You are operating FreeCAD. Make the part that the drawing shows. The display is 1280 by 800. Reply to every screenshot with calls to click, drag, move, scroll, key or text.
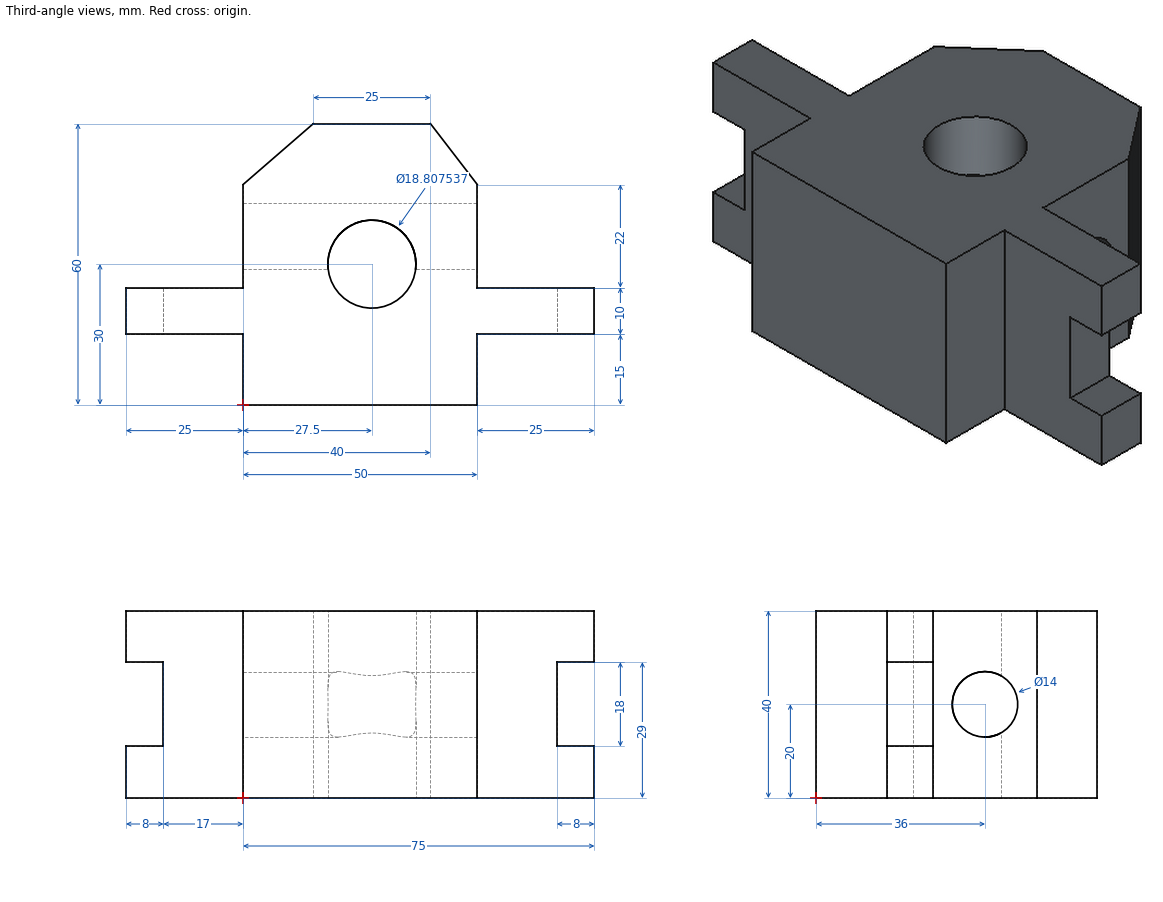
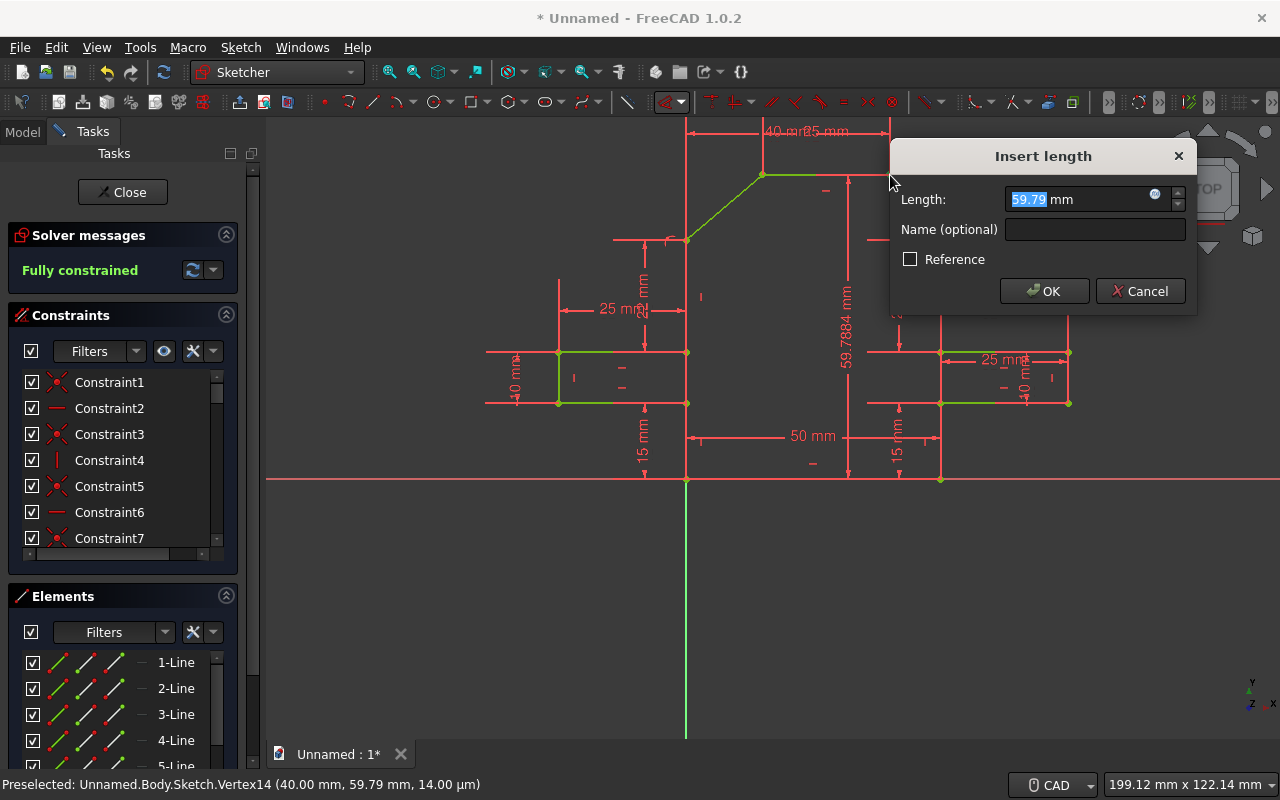
text(60)
key(Return)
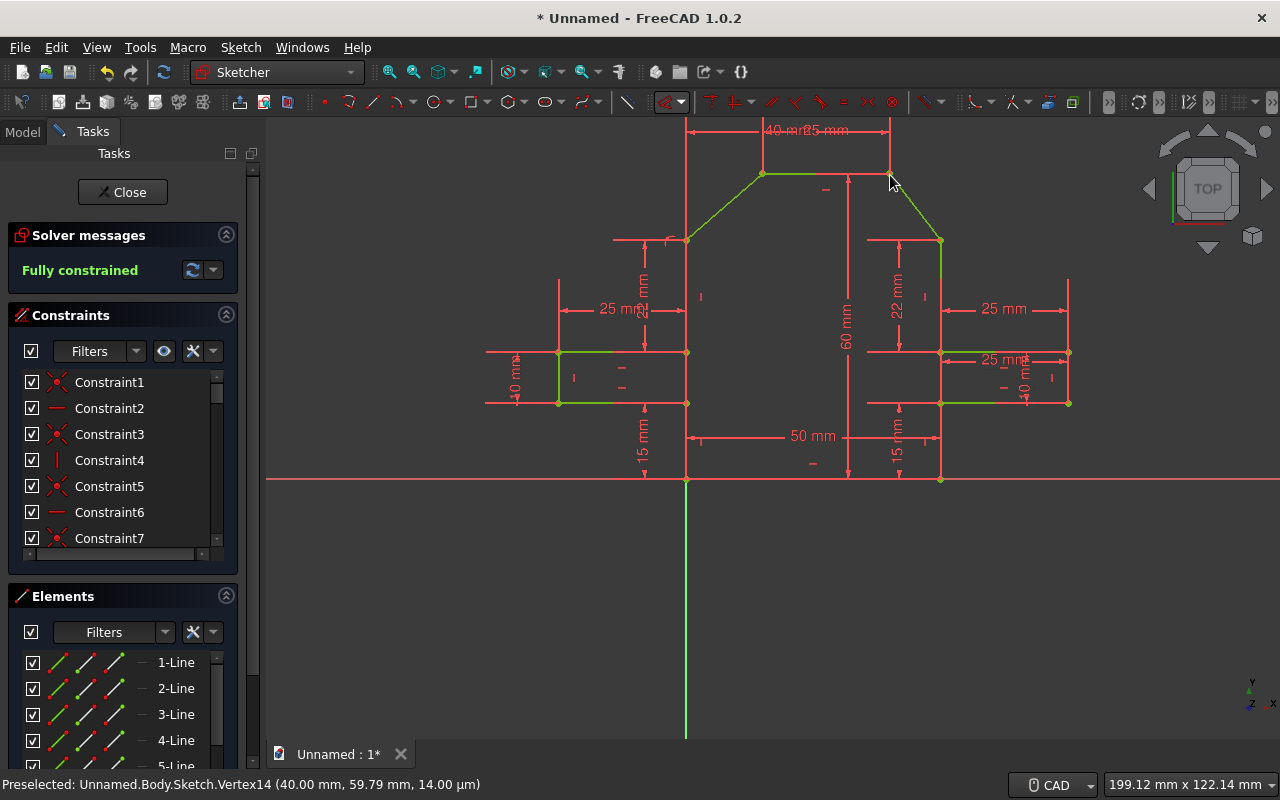
click(123, 192)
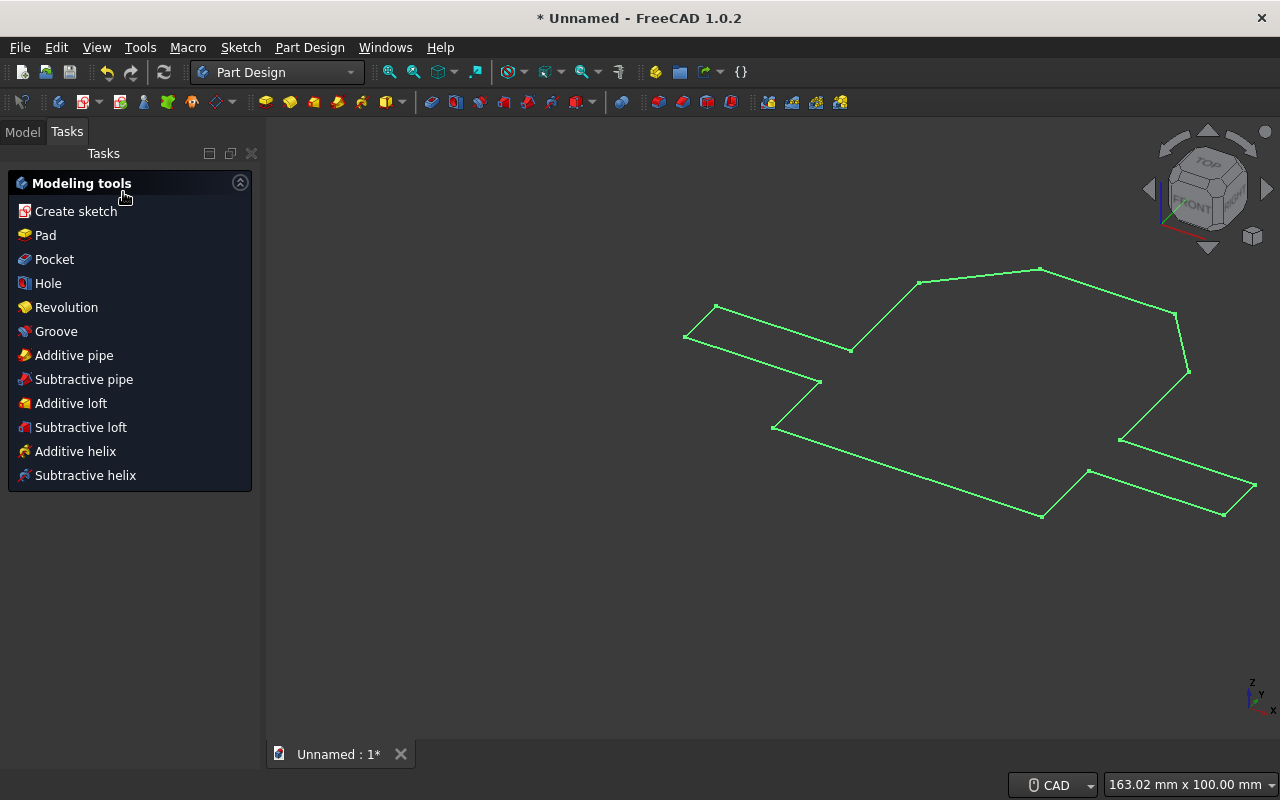
click(266, 102)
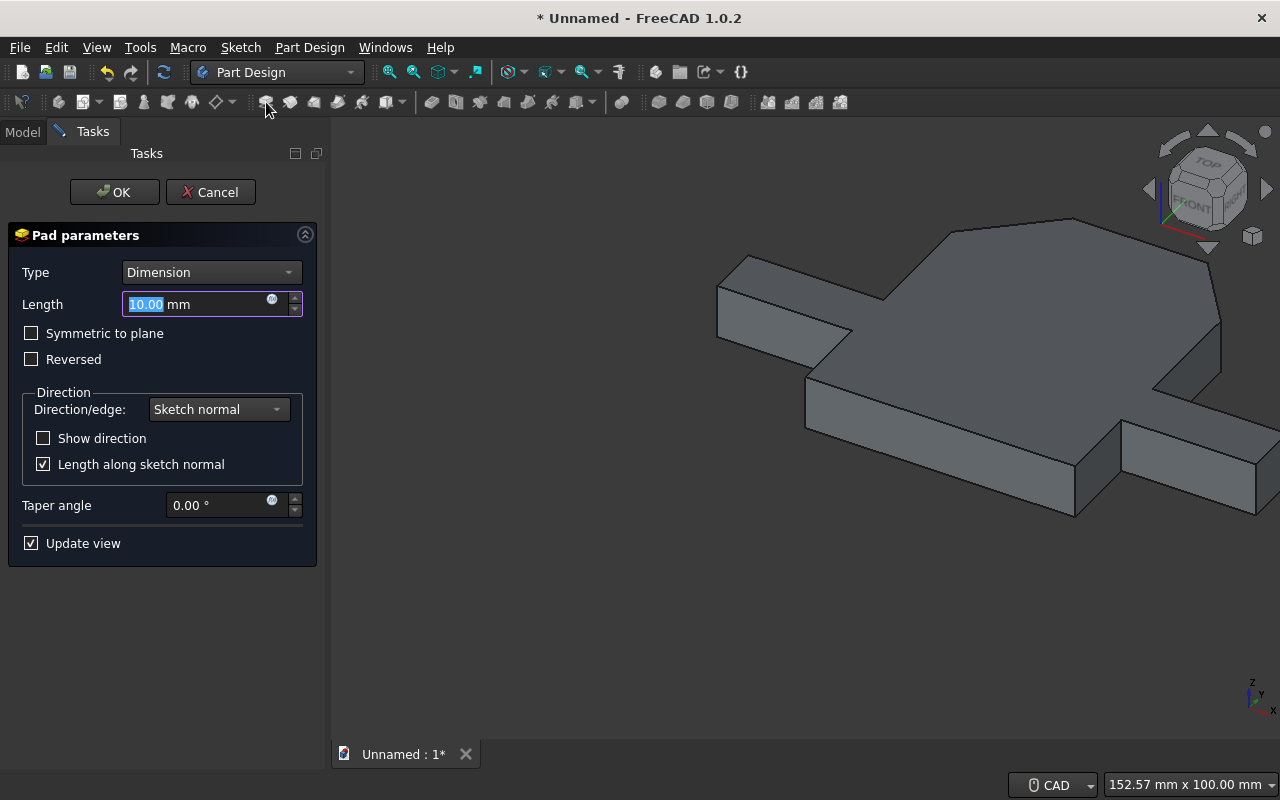
text(40)
key(Tab)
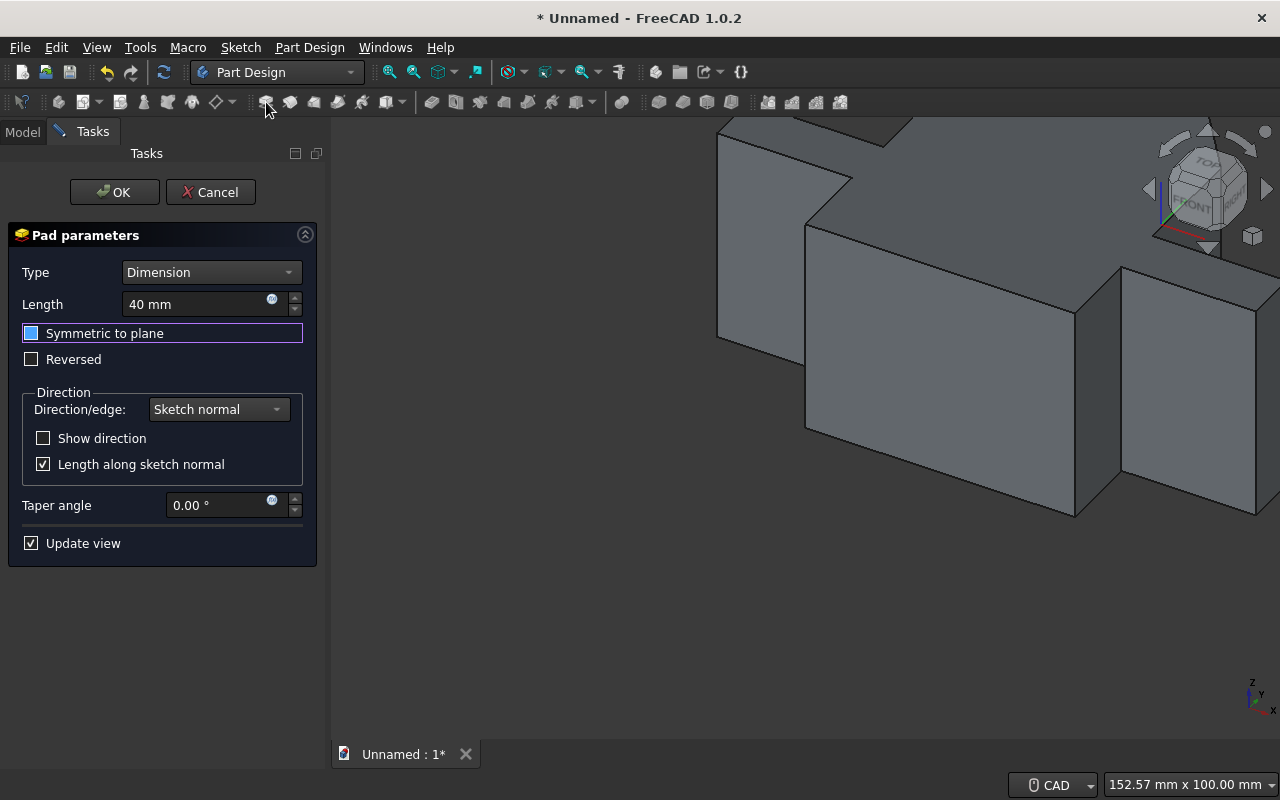
click(115, 192)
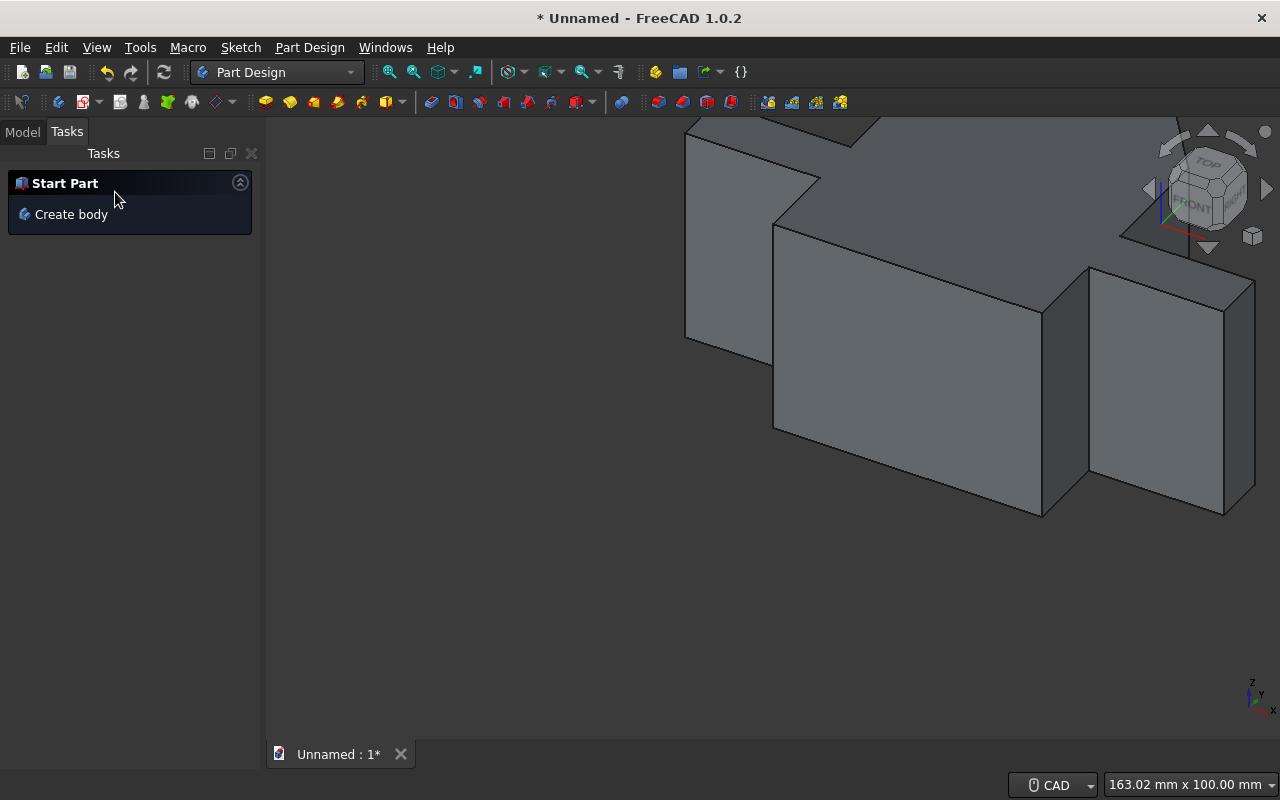
key(v)
key(f)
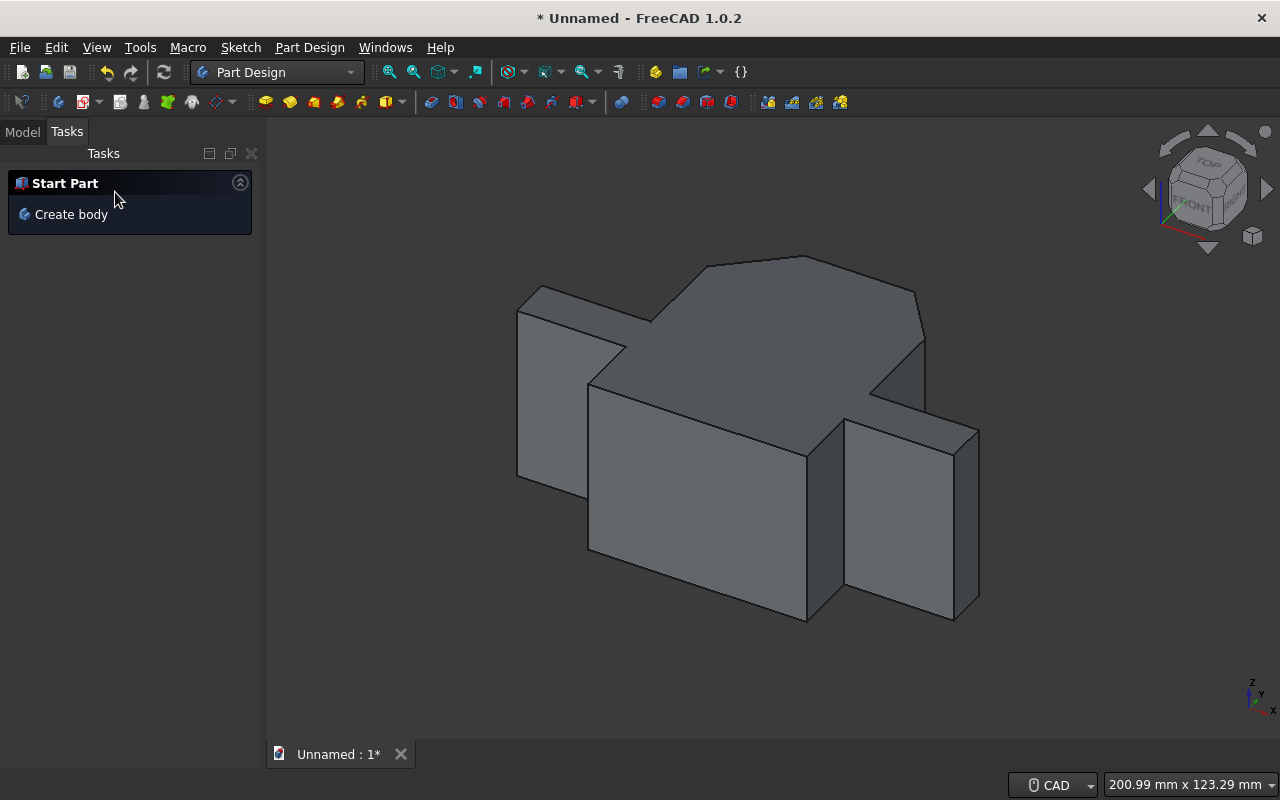
click(773, 344)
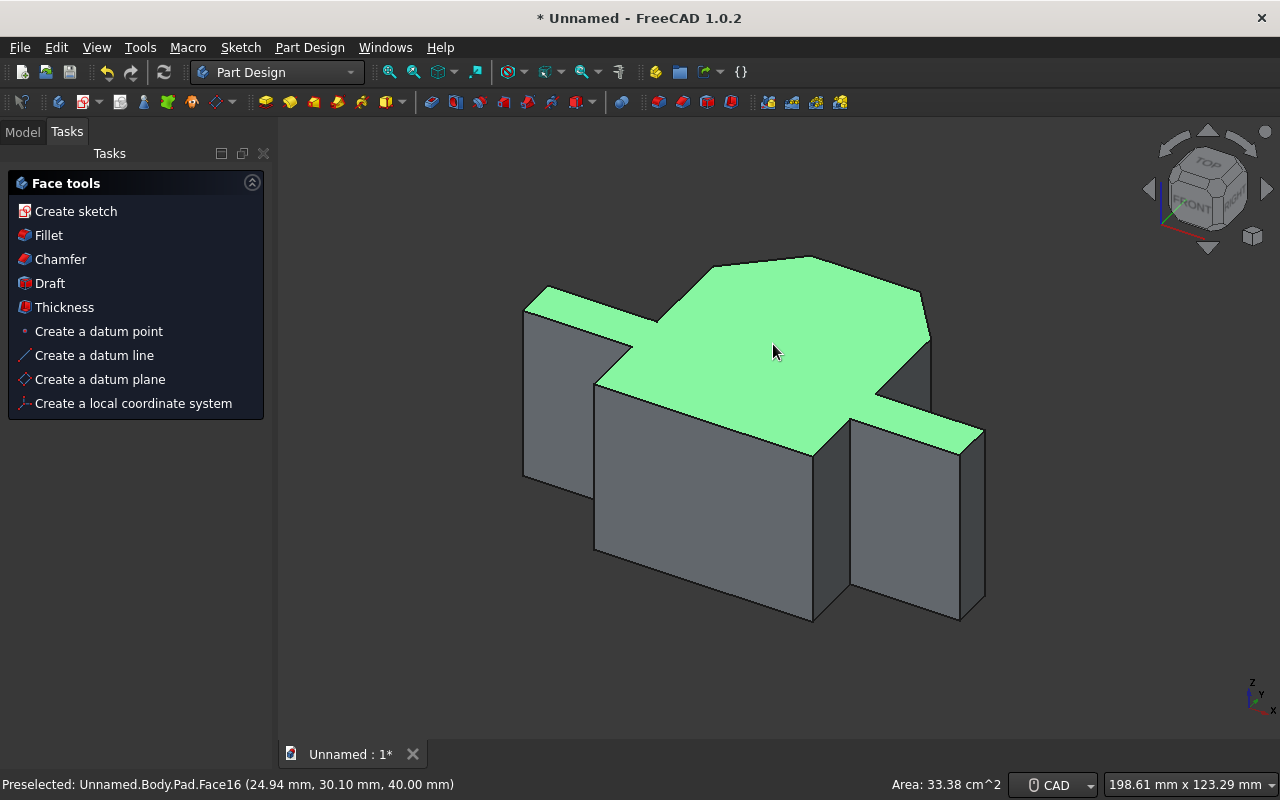
click(84, 102)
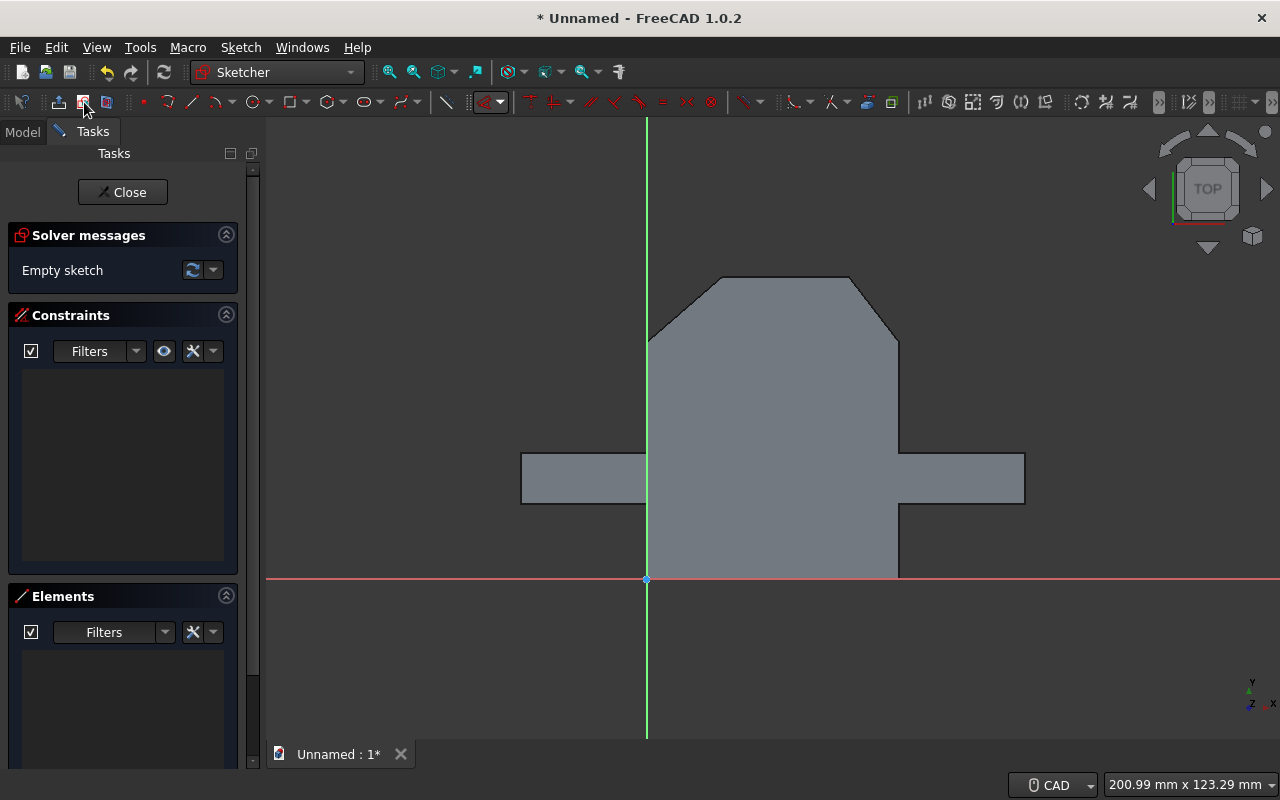
scroll(783, 543, up, 3)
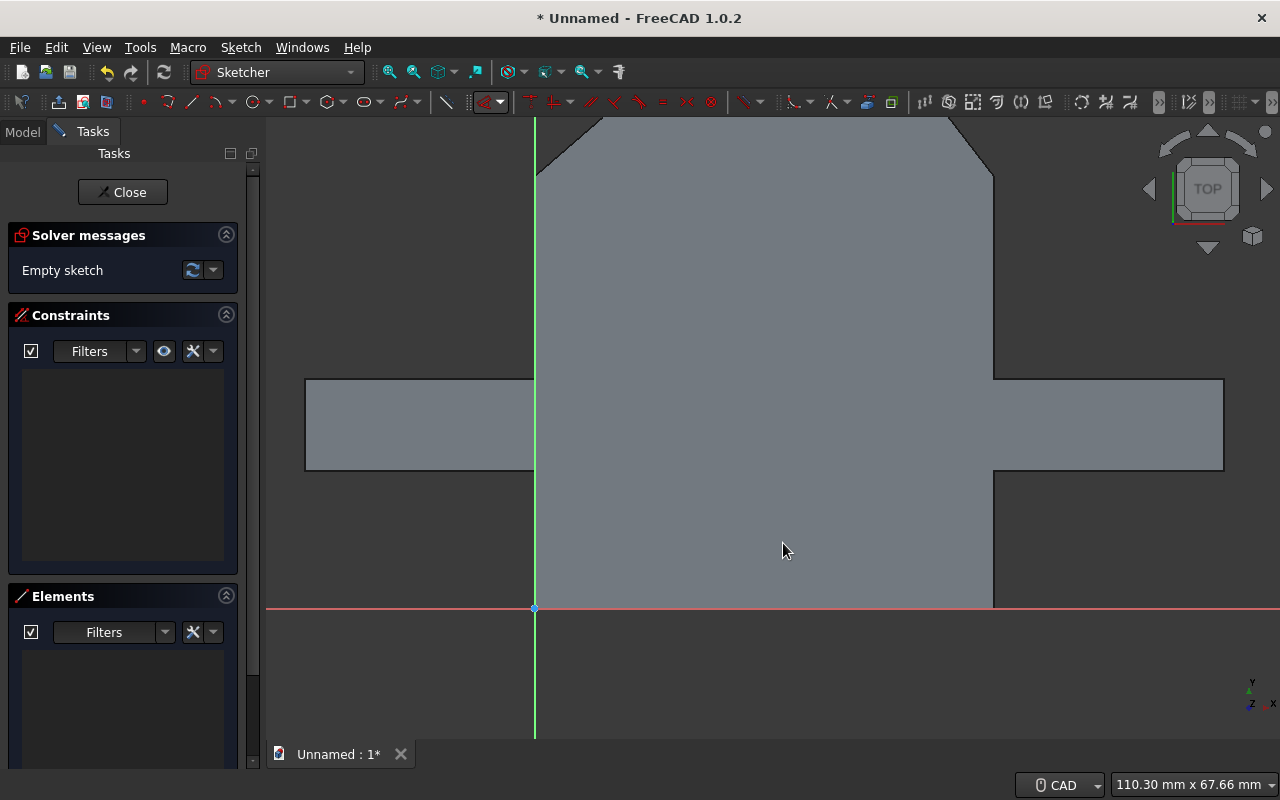
click(254, 102)